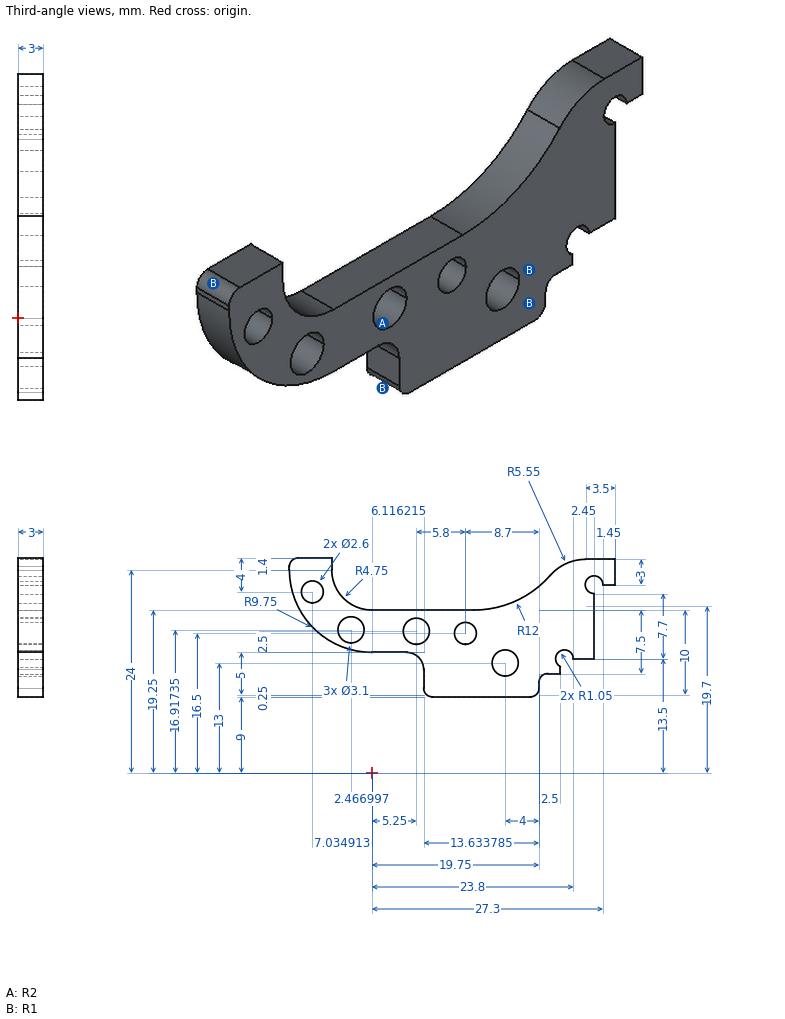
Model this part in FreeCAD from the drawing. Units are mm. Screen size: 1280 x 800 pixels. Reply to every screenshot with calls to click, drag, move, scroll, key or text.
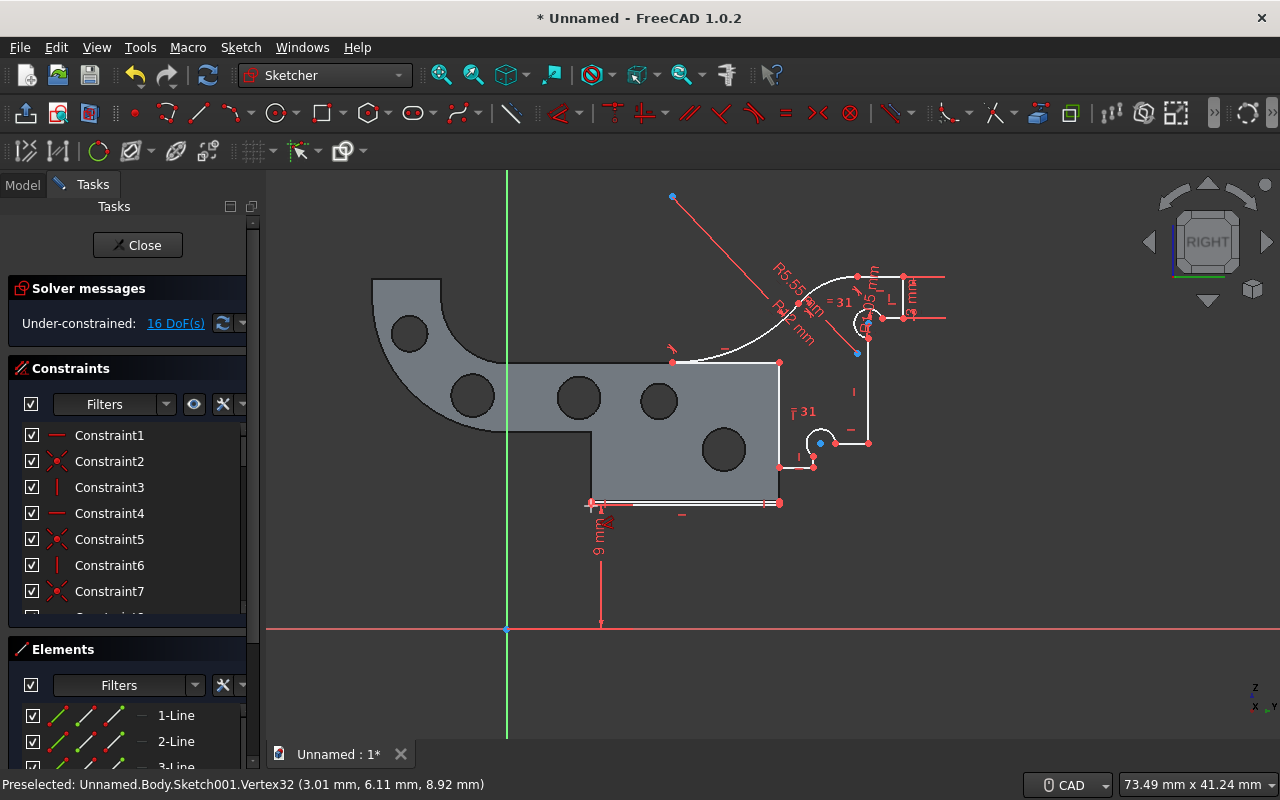
click(868, 412)
click(902, 391)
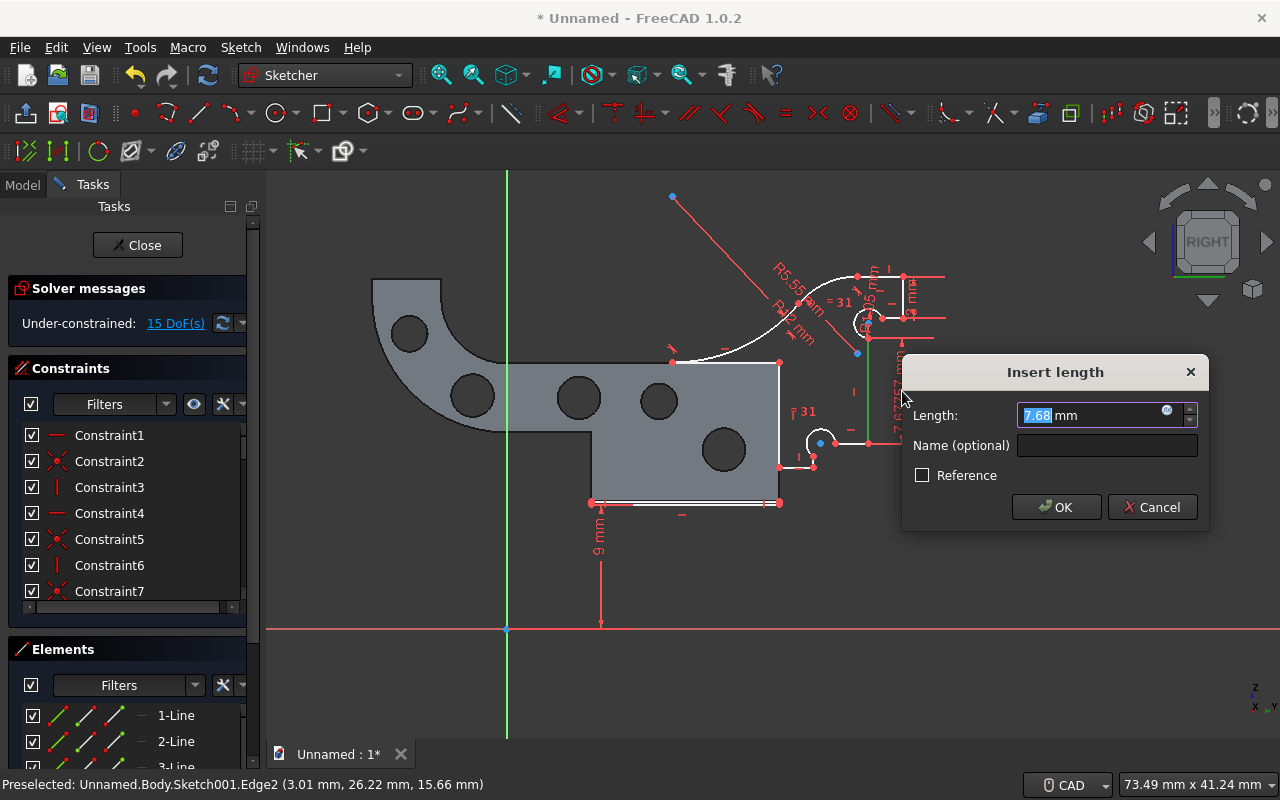
text(7.7)
key(Return)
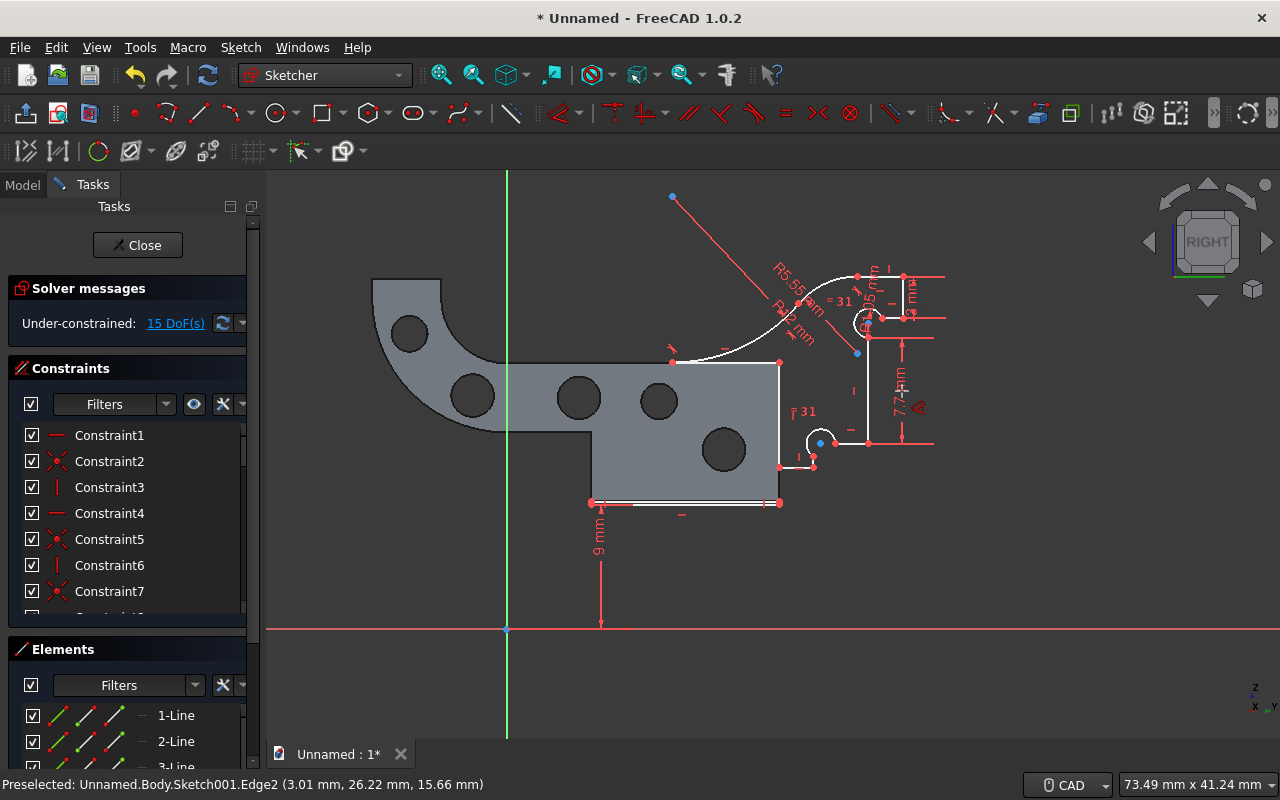
click(890, 277)
click(880, 243)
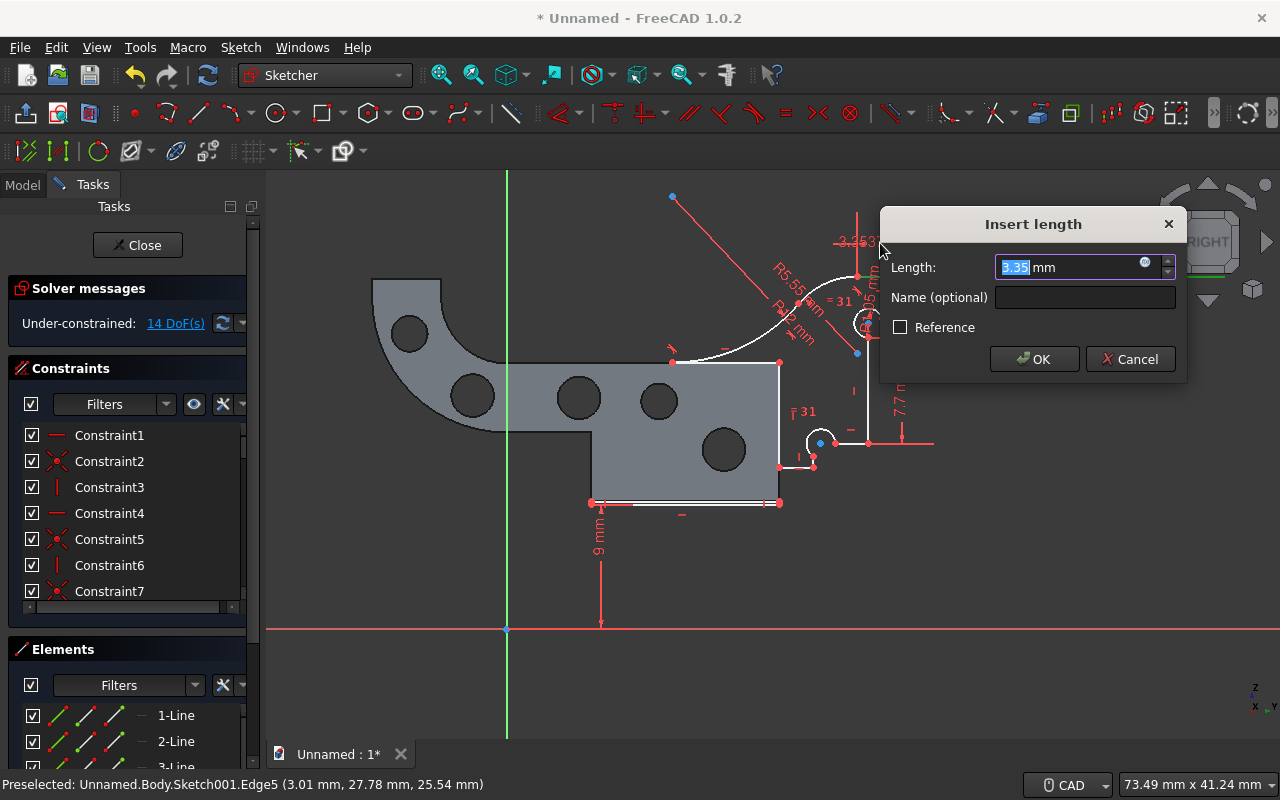
text(3.5)
key(Return)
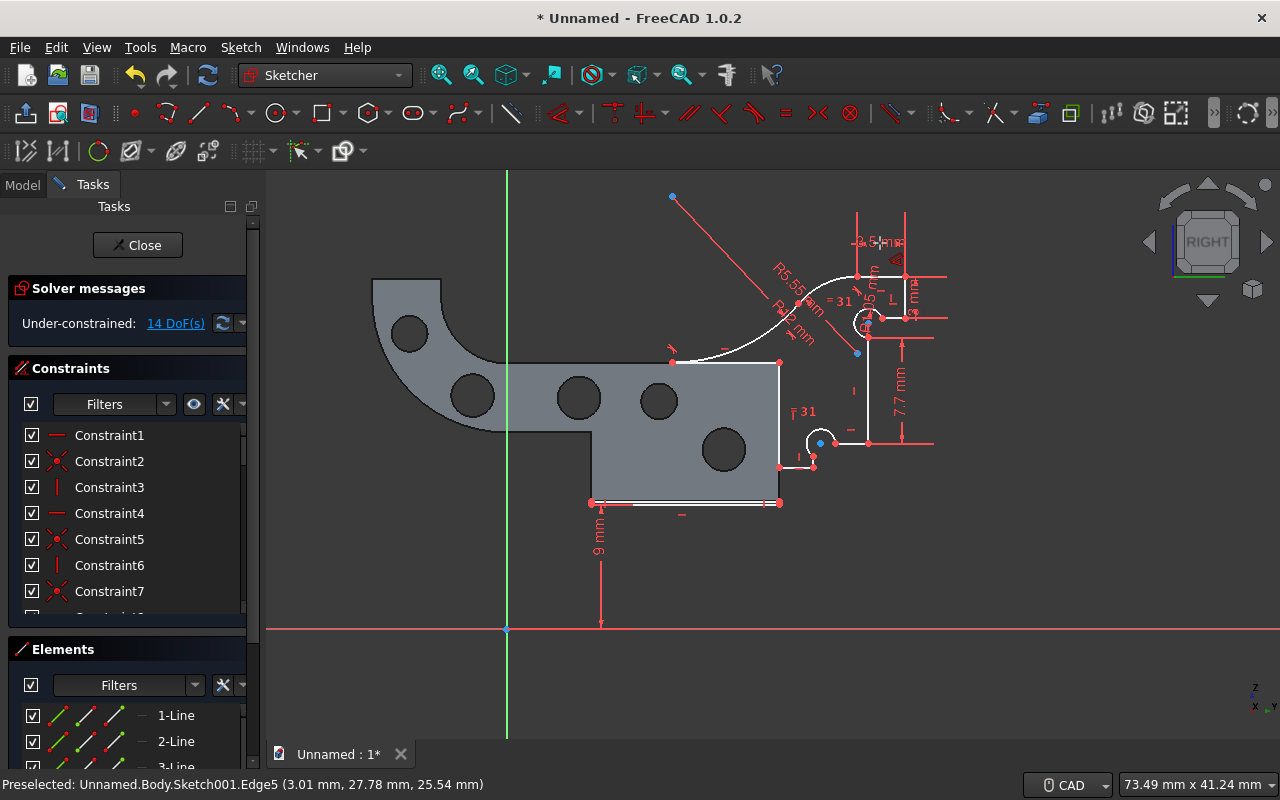
click(779, 394)
click(813, 415)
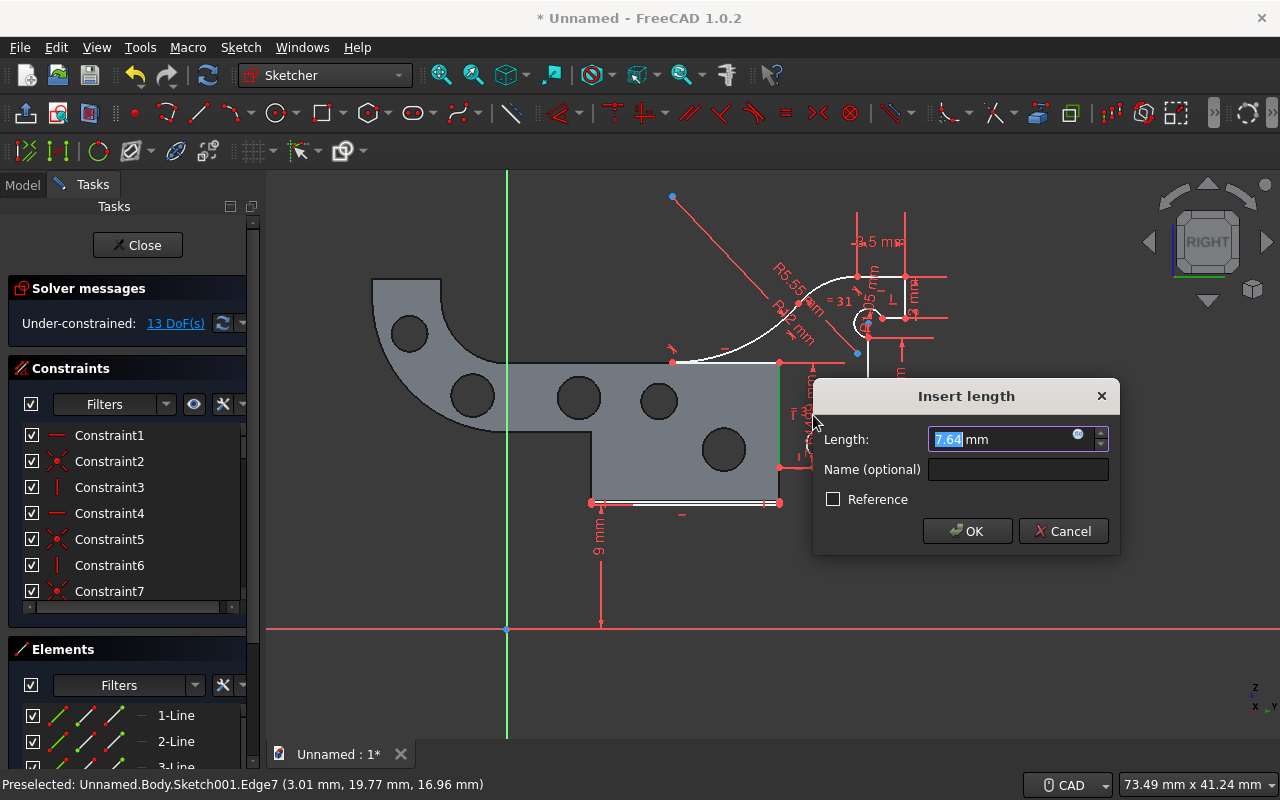
text(7.5)
key(Return)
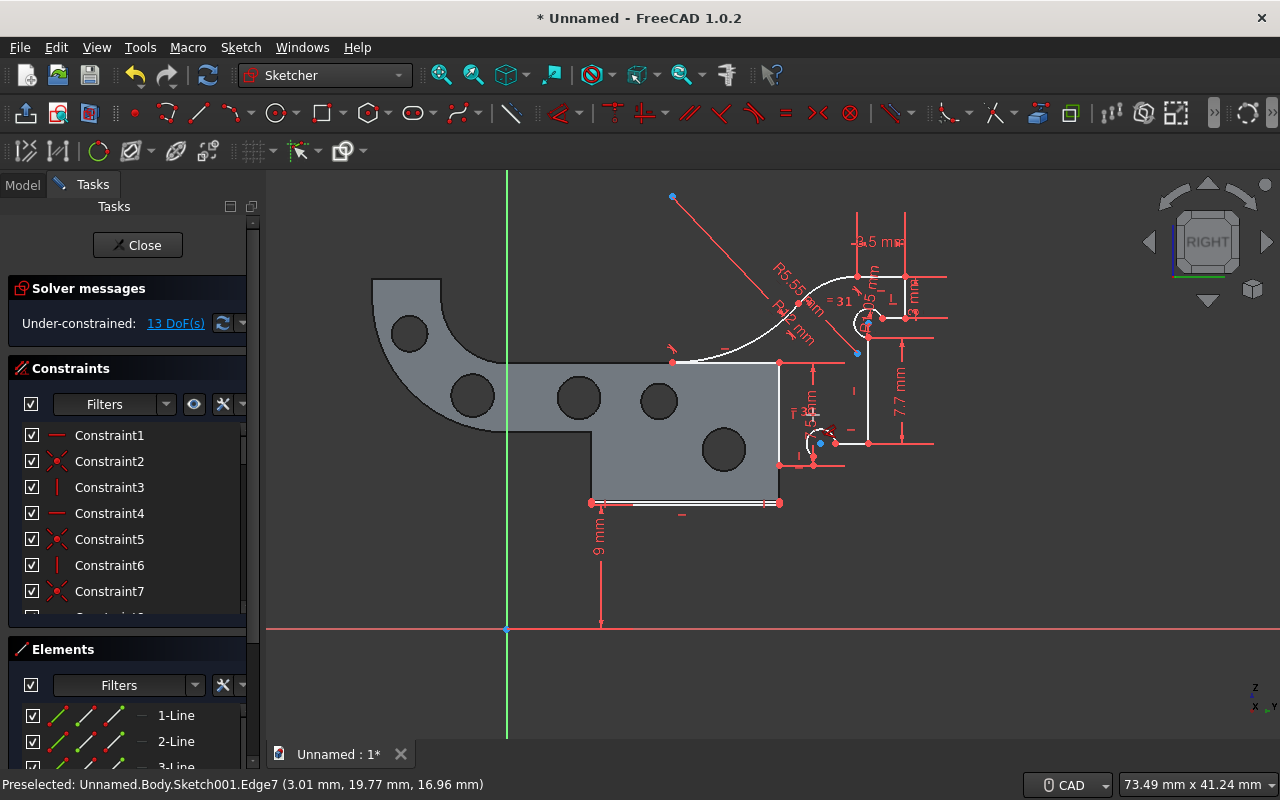
scroll(790, 466, up, 2)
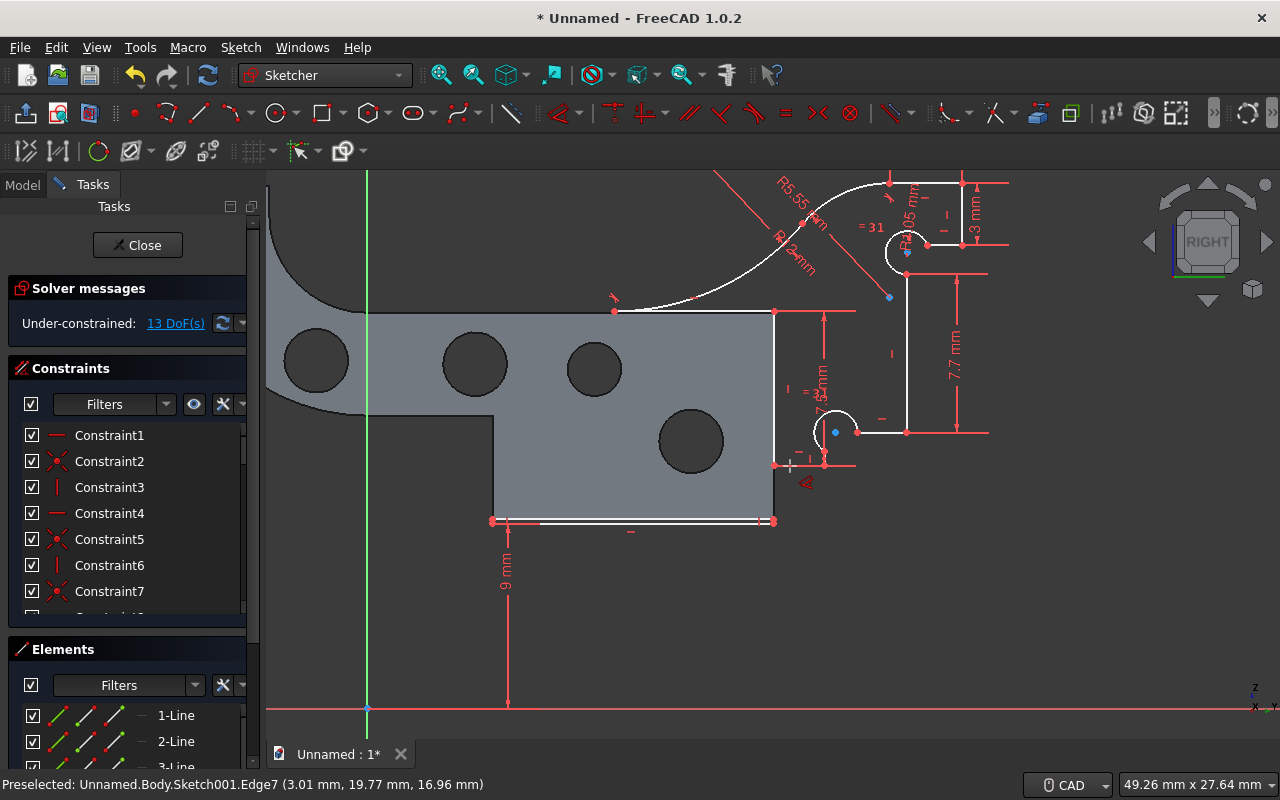
click(789, 466)
click(799, 500)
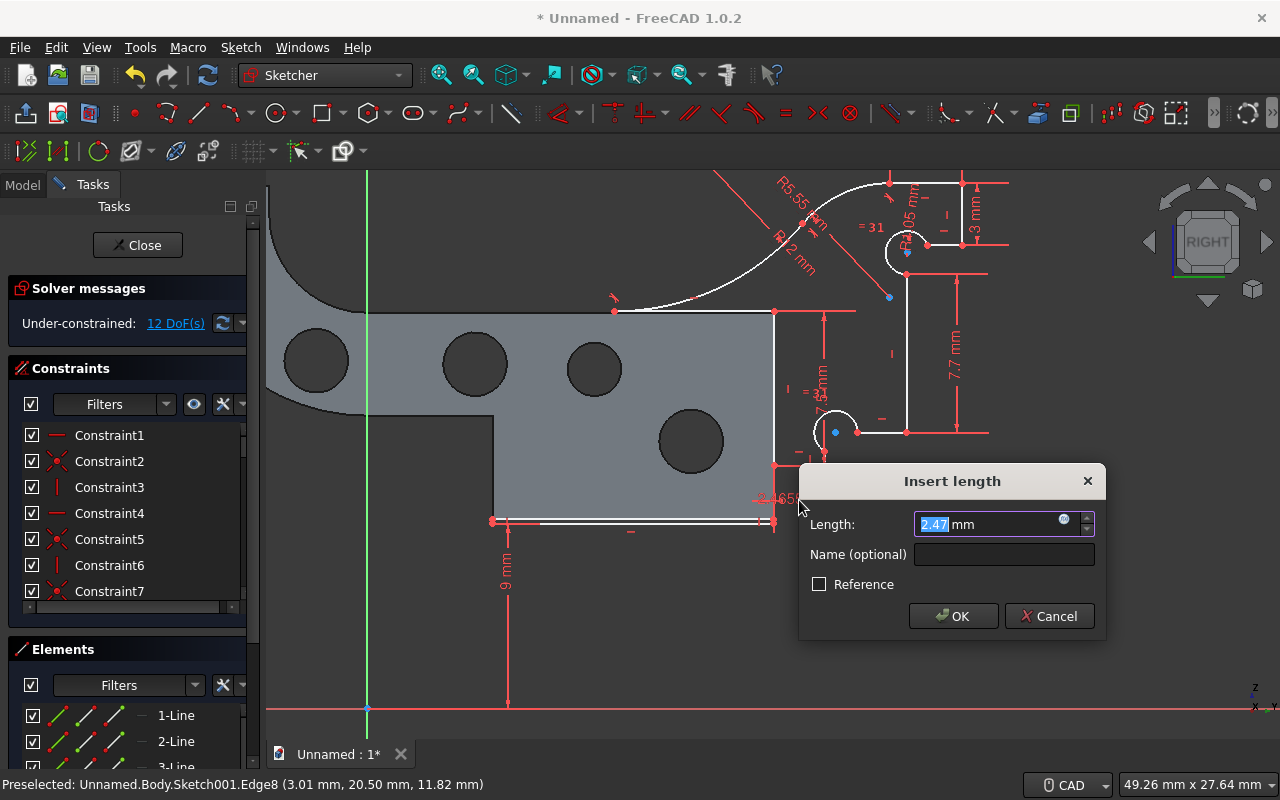
text(2.5)
key(Return)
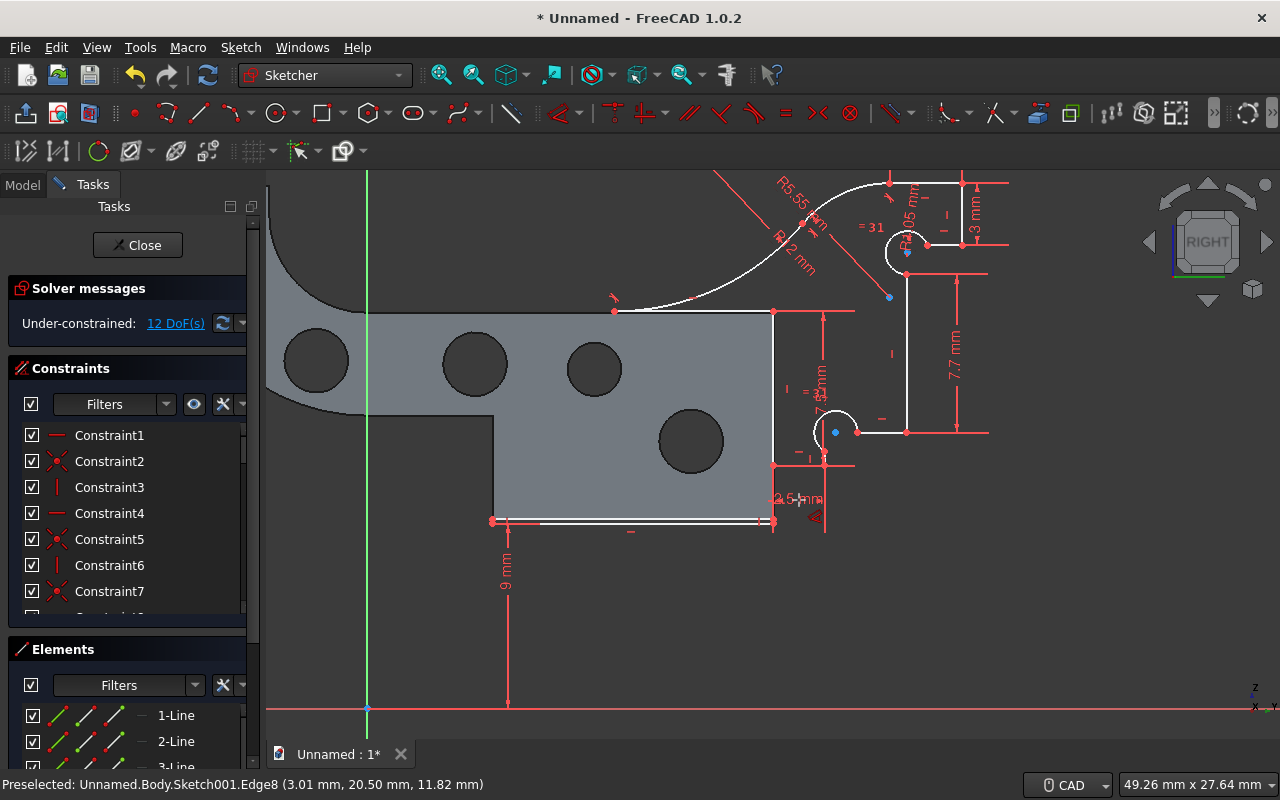
click(872, 433)
click(882, 467)